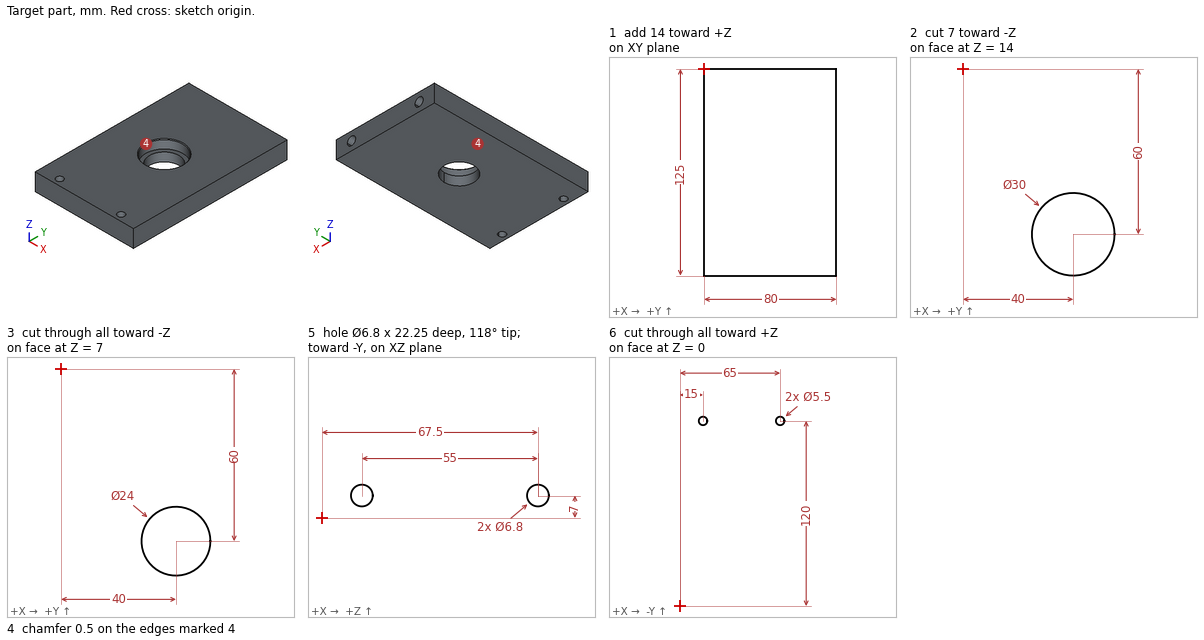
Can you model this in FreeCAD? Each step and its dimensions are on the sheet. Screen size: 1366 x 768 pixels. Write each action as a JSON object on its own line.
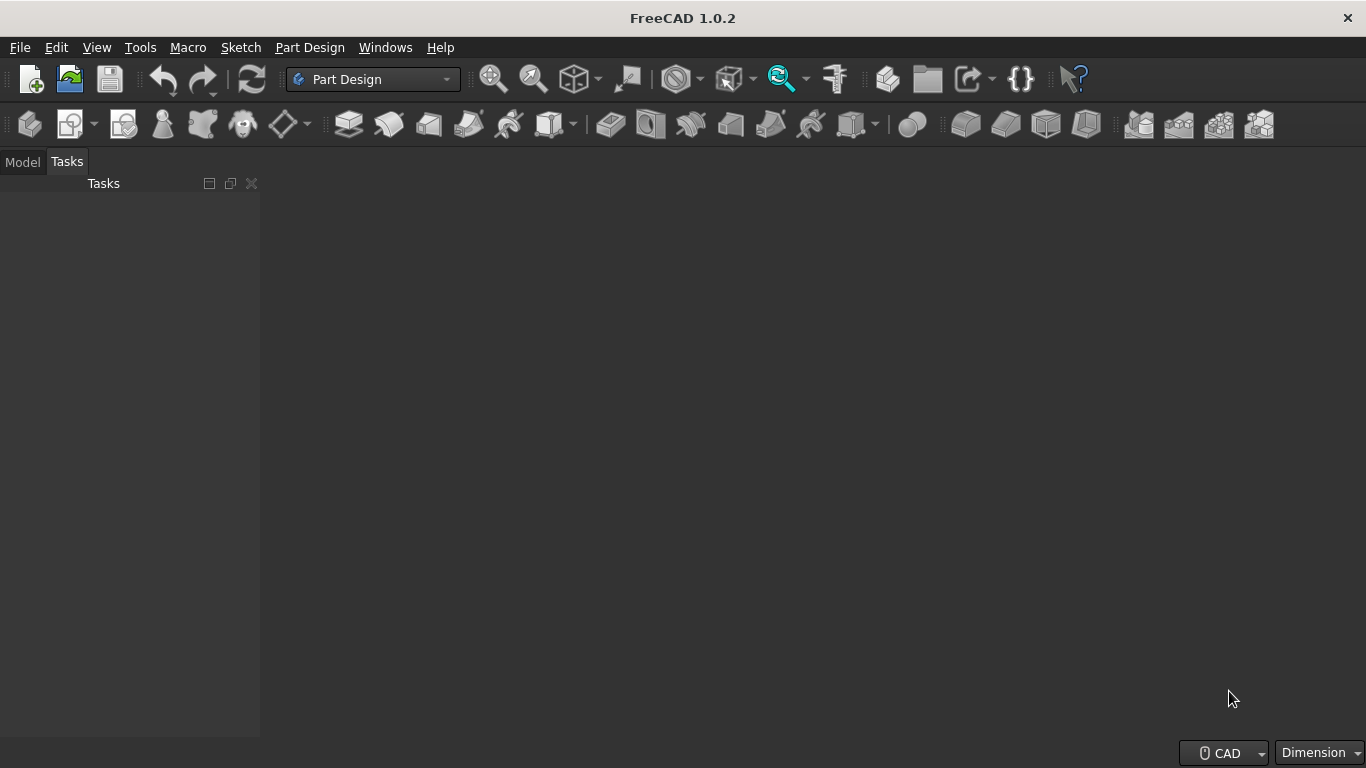
{"action": "left_click", "coordinate": [30, 80]}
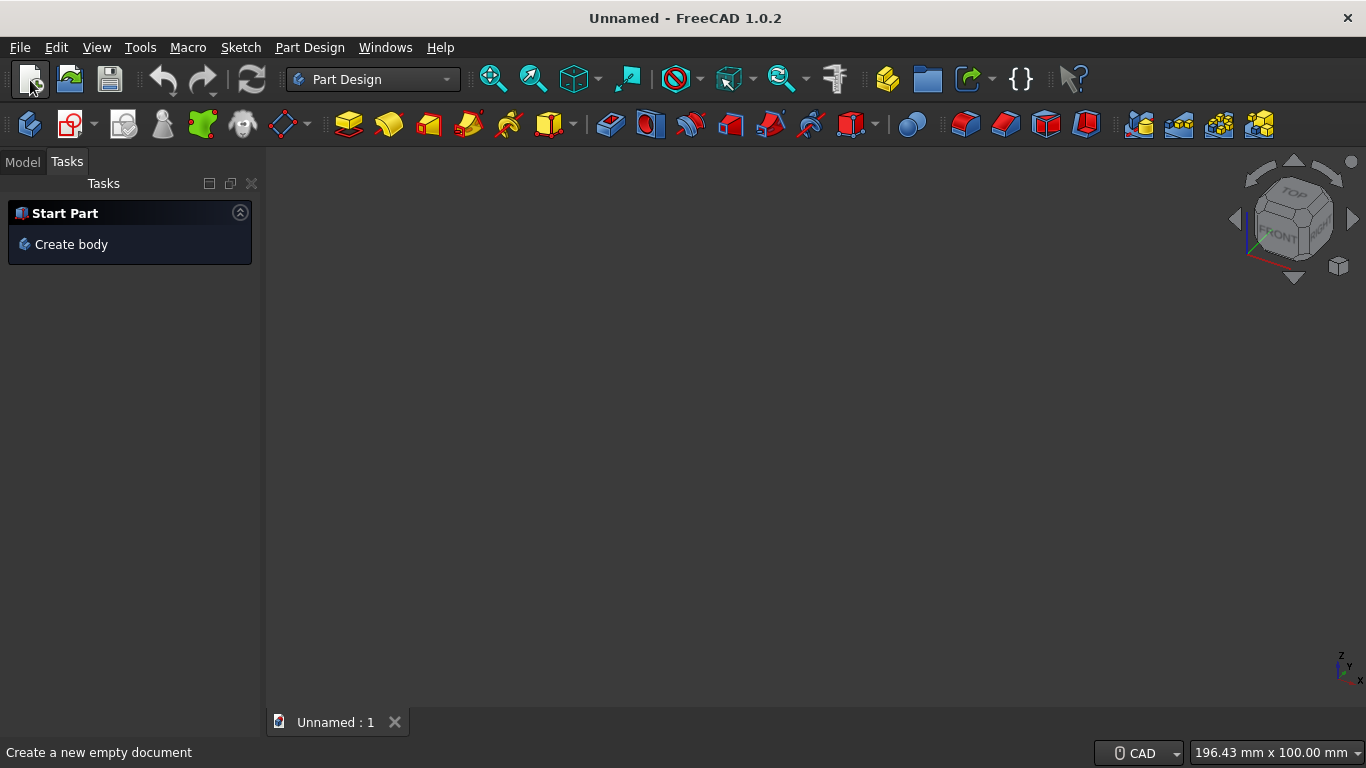
{"action": "left_click", "coordinate": [70, 124]}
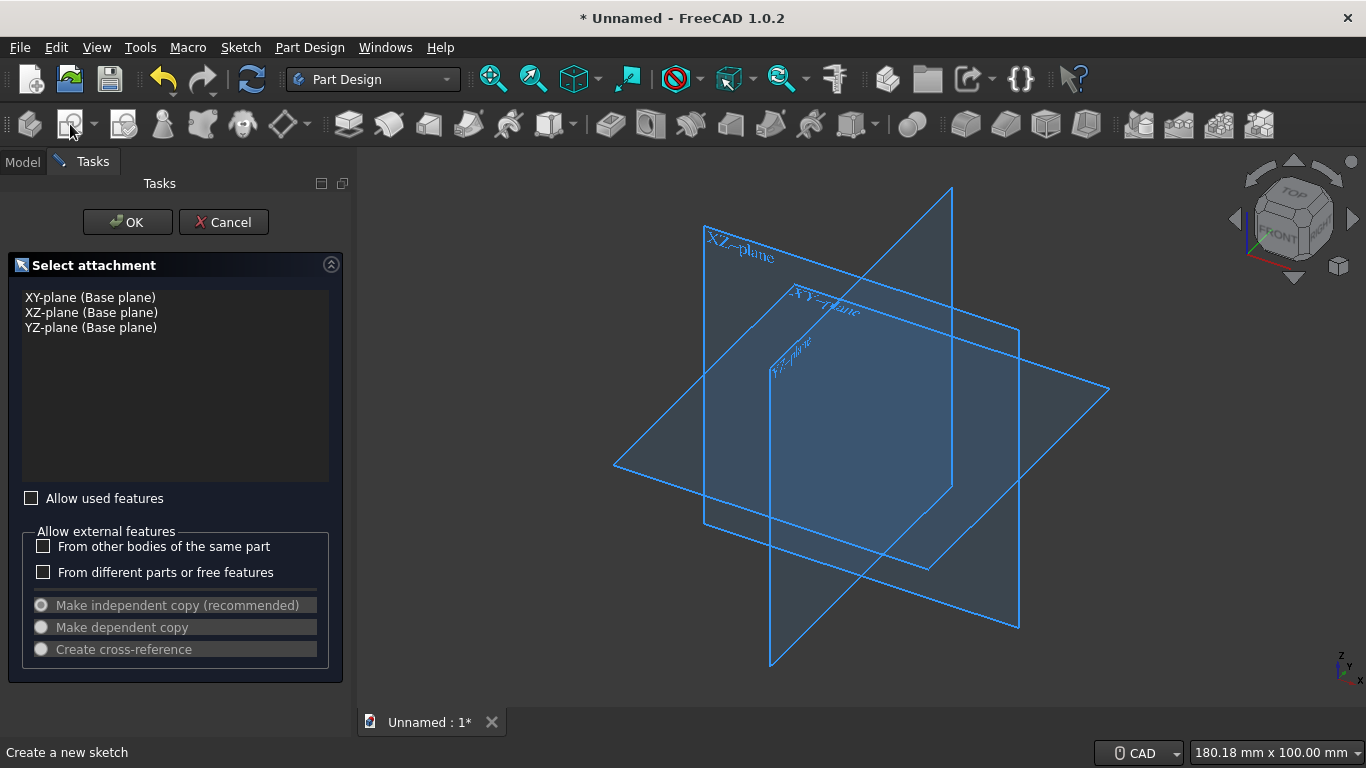
{"action": "left_click", "coordinate": [82, 298]}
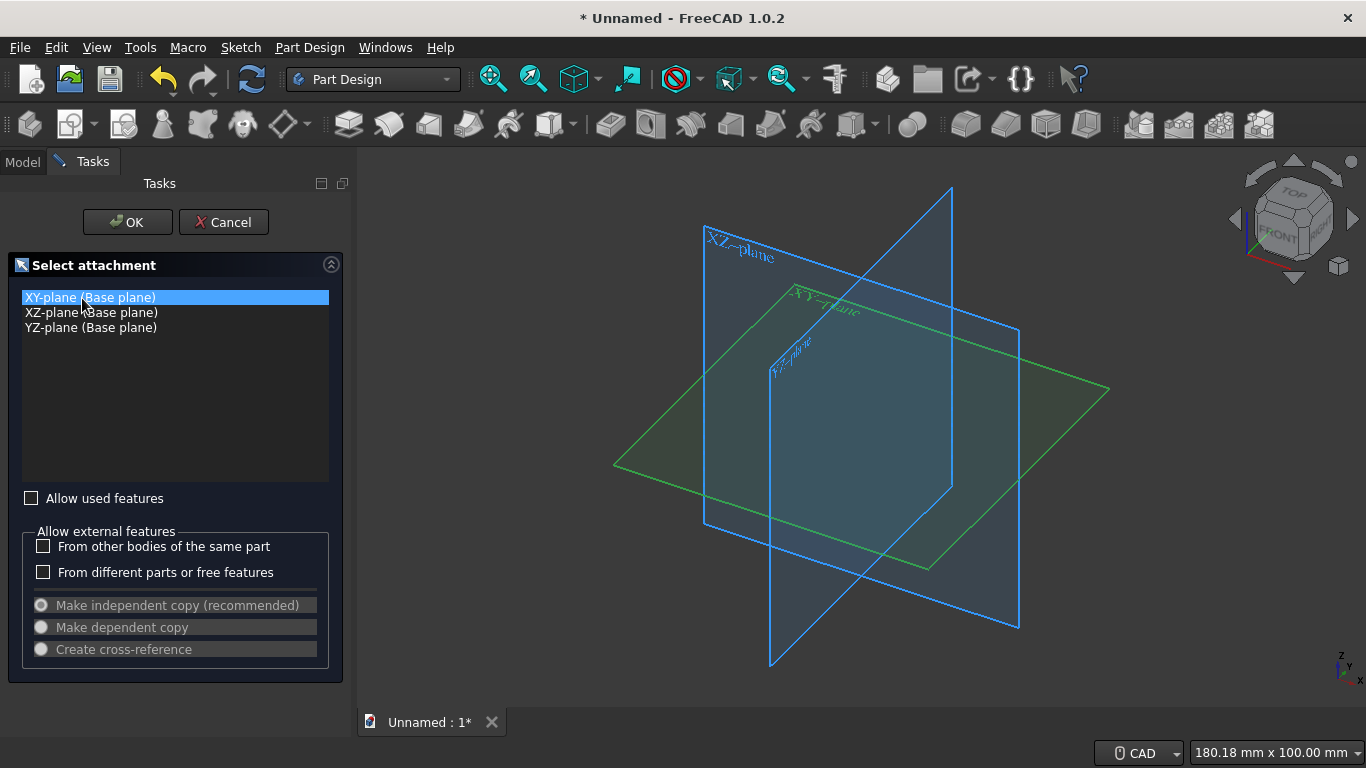
{"action": "left_click", "coordinate": [128, 222]}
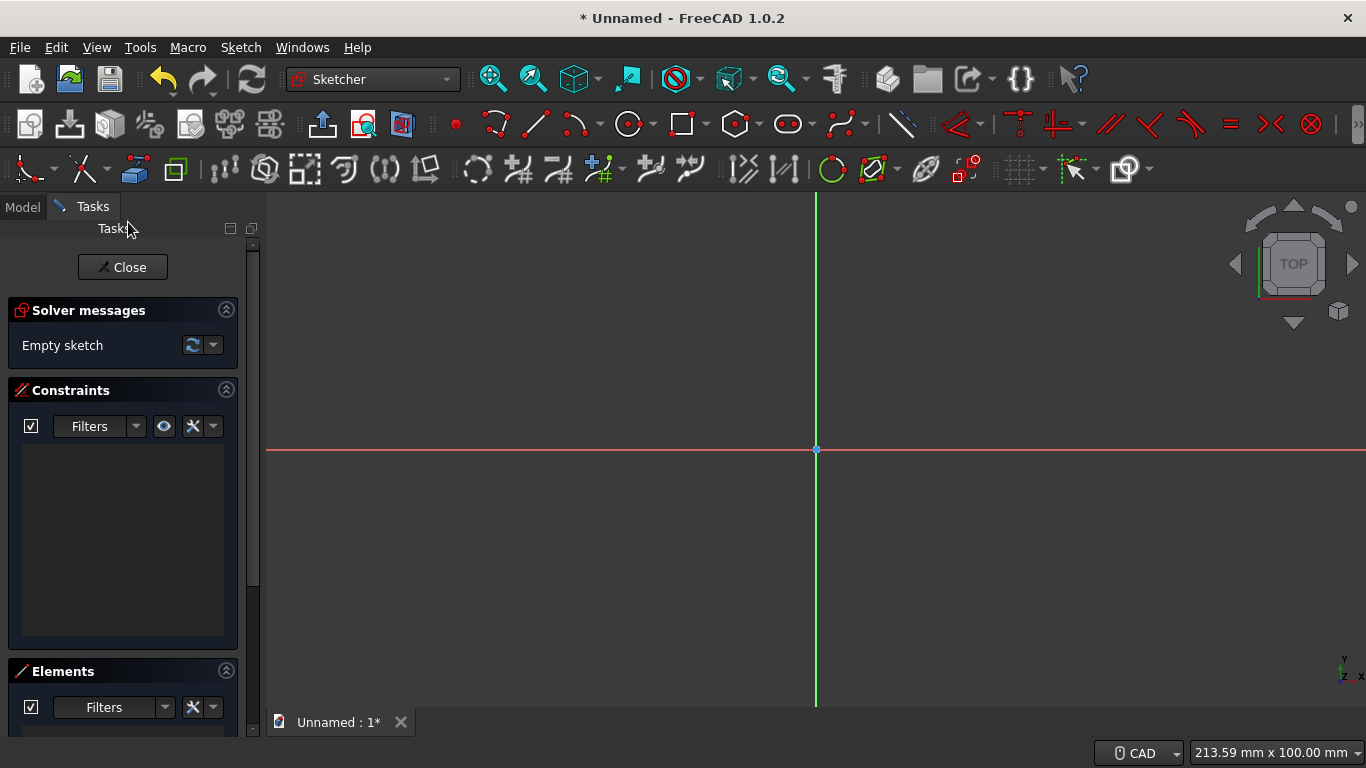
{"action": "scroll", "coordinate": [524, 220], "scroll_direction": "down", "scroll_amount": 4}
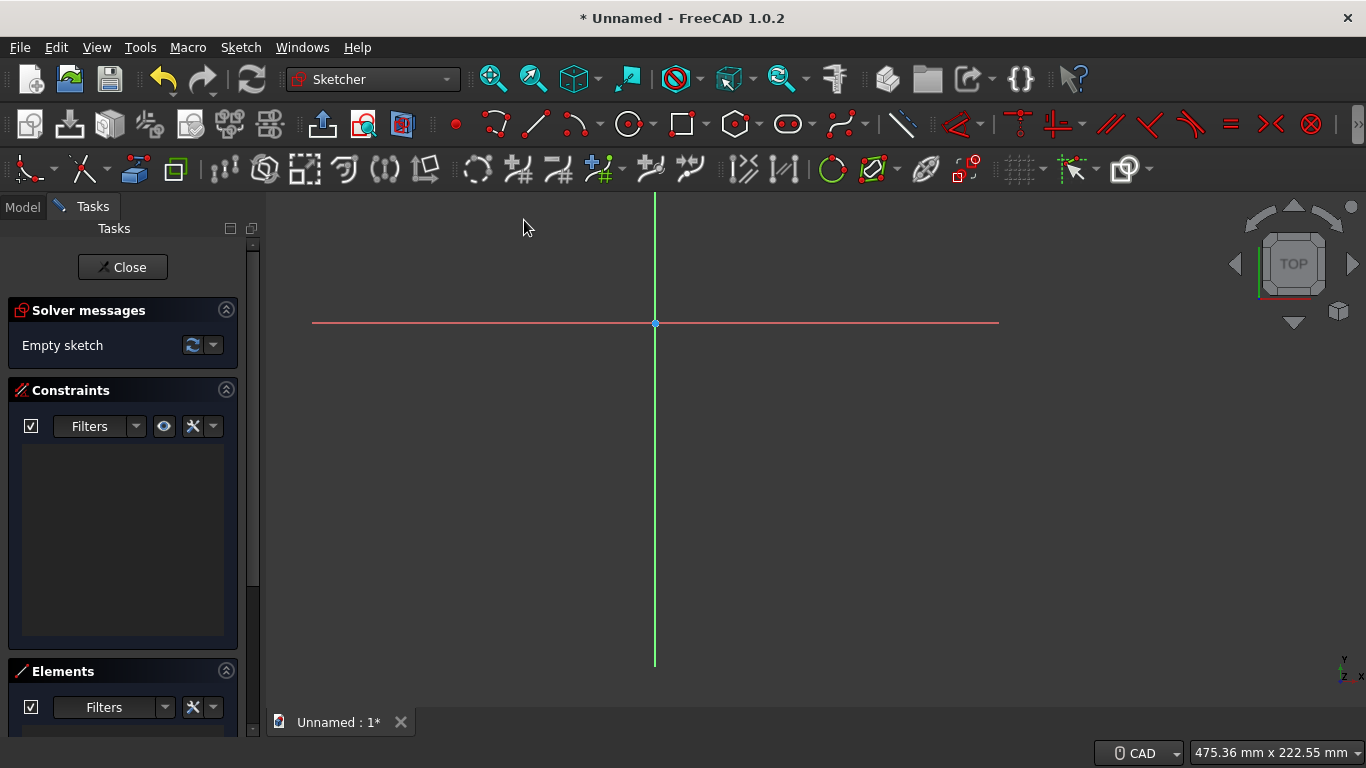
{"action": "left_click", "coordinate": [682, 124]}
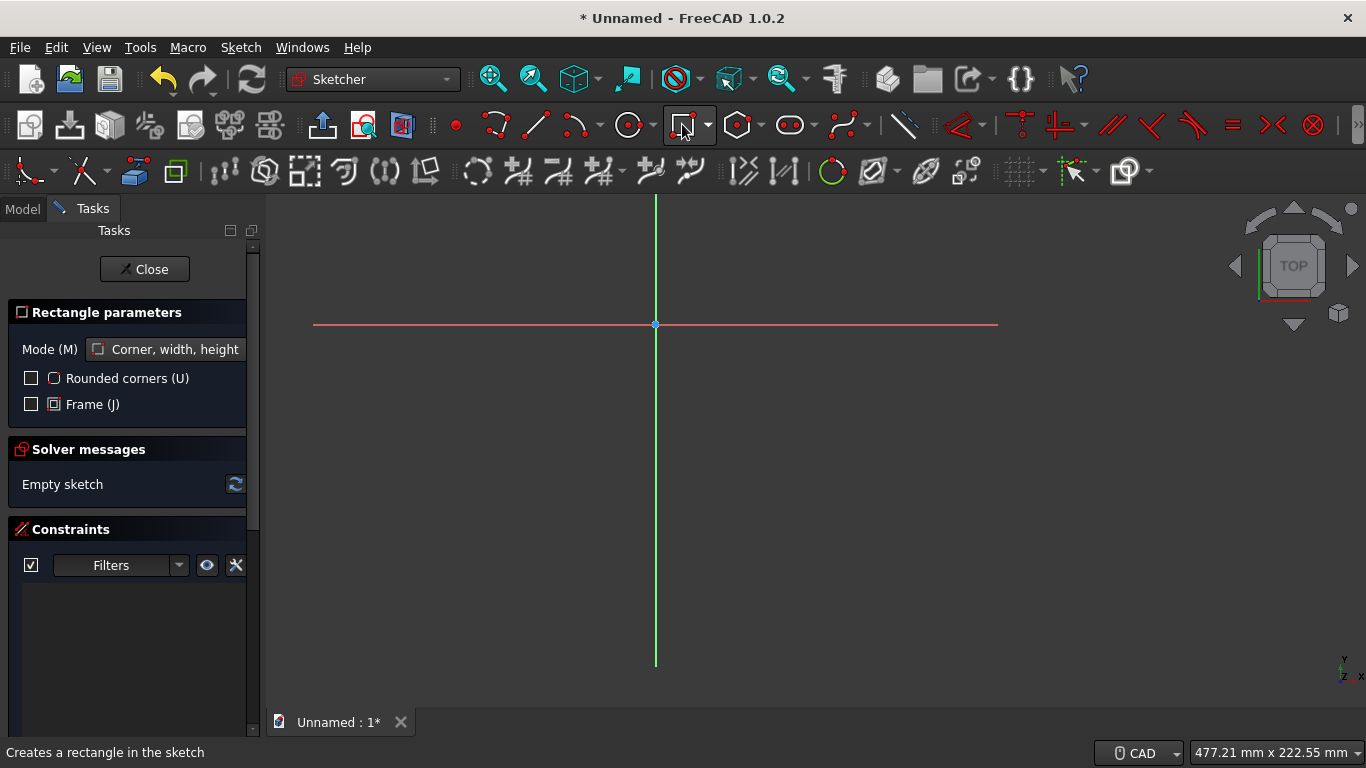
{"action": "left_click", "coordinate": [656, 325]}
{"action": "left_click", "coordinate": [840, 613]}
{"action": "key", "text": "Escape"}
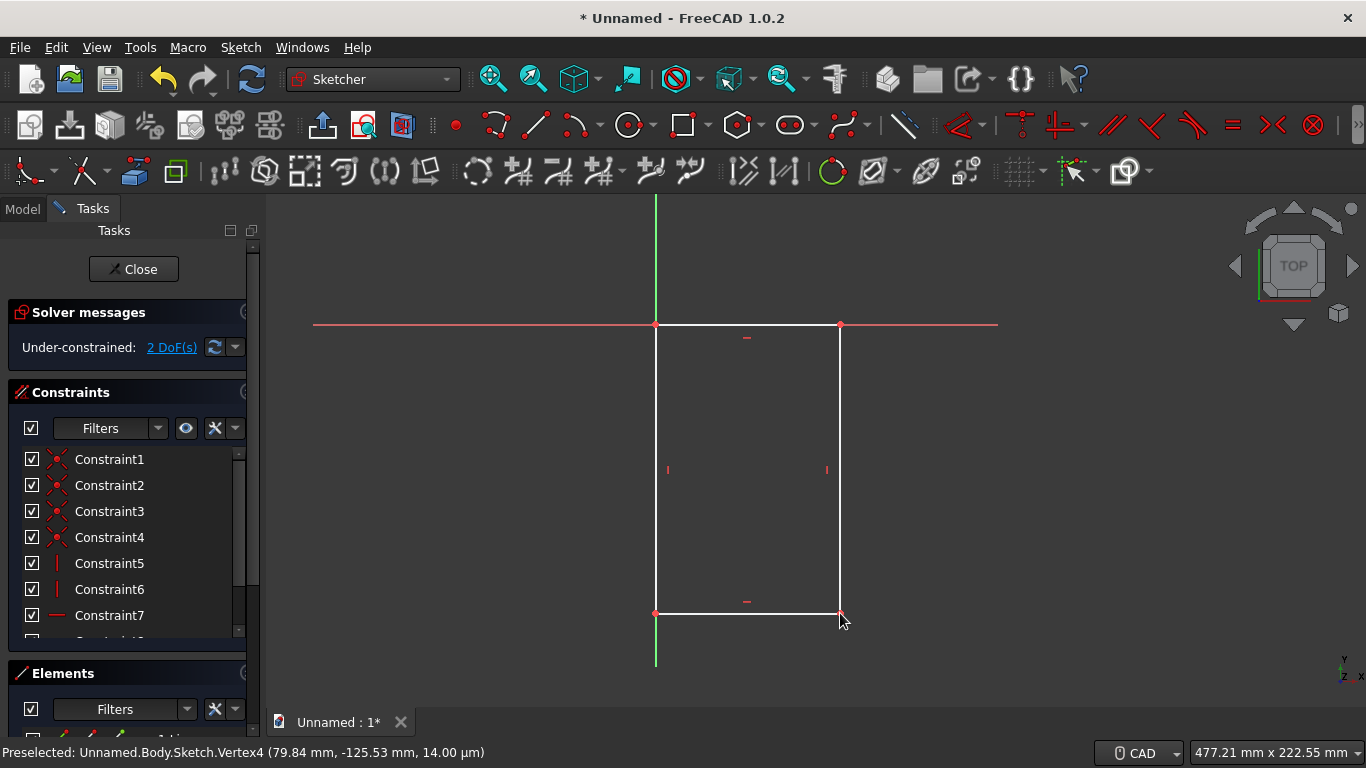
{"action": "left_click", "coordinate": [958, 126]}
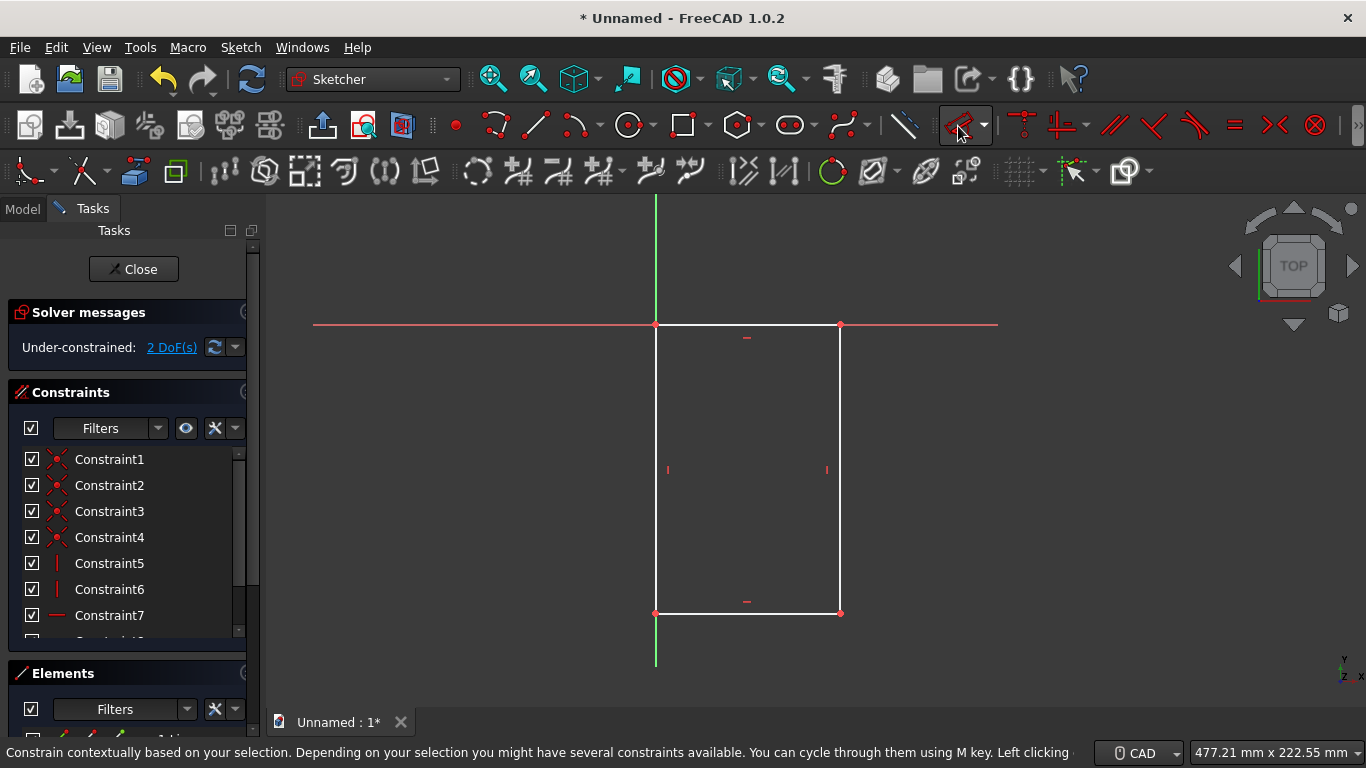
{"action": "left_click", "coordinate": [711, 614]}
{"action": "left_click", "coordinate": [748, 648]}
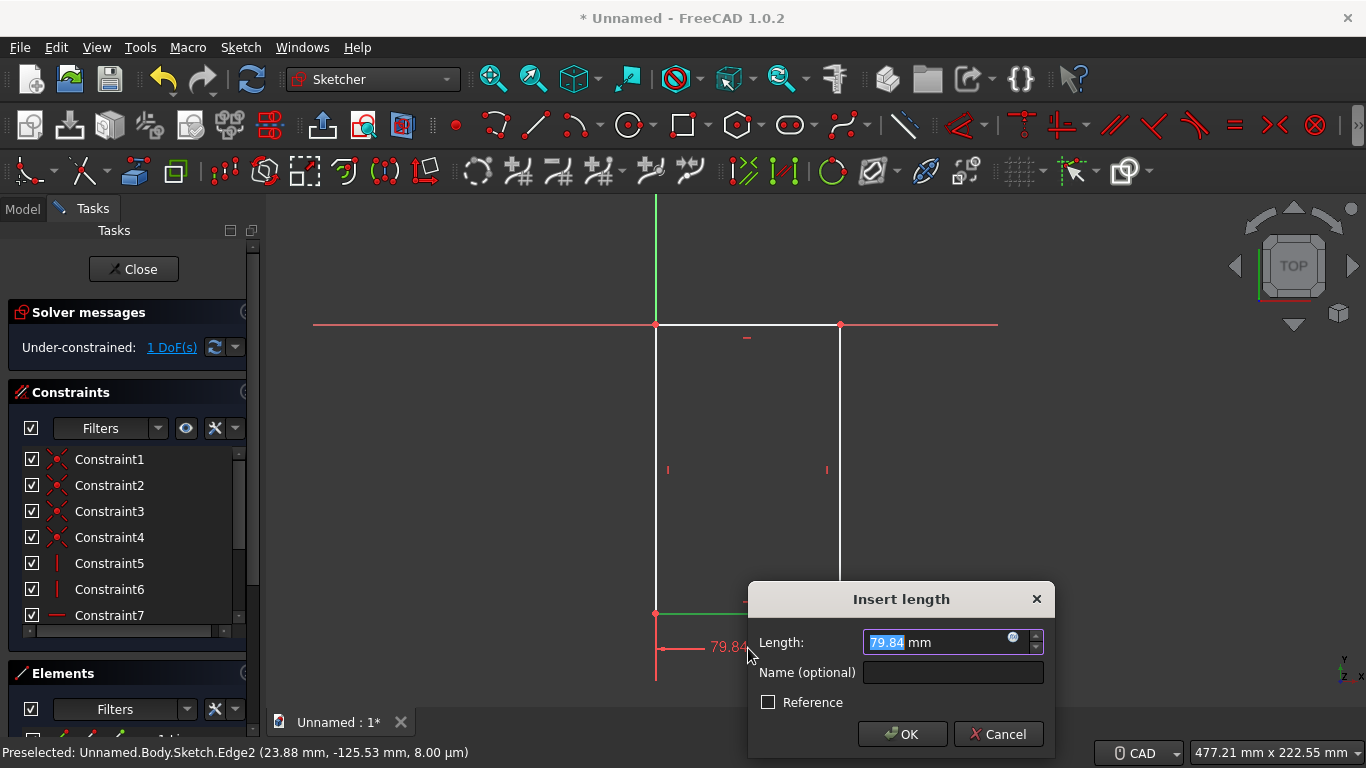
{"action": "type", "text": "80"}
{"action": "key", "text": "Return"}